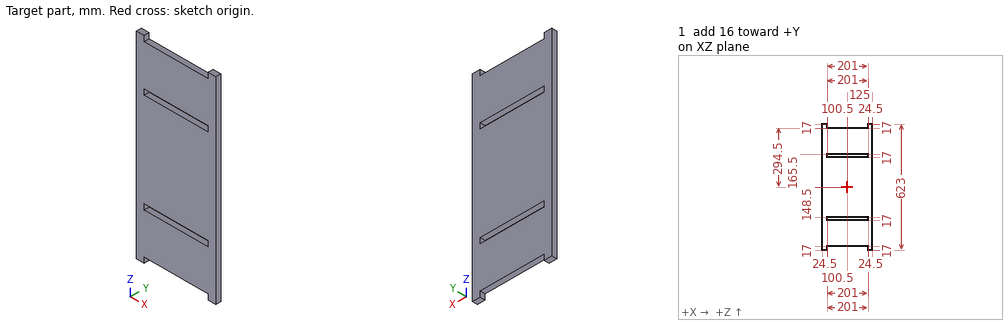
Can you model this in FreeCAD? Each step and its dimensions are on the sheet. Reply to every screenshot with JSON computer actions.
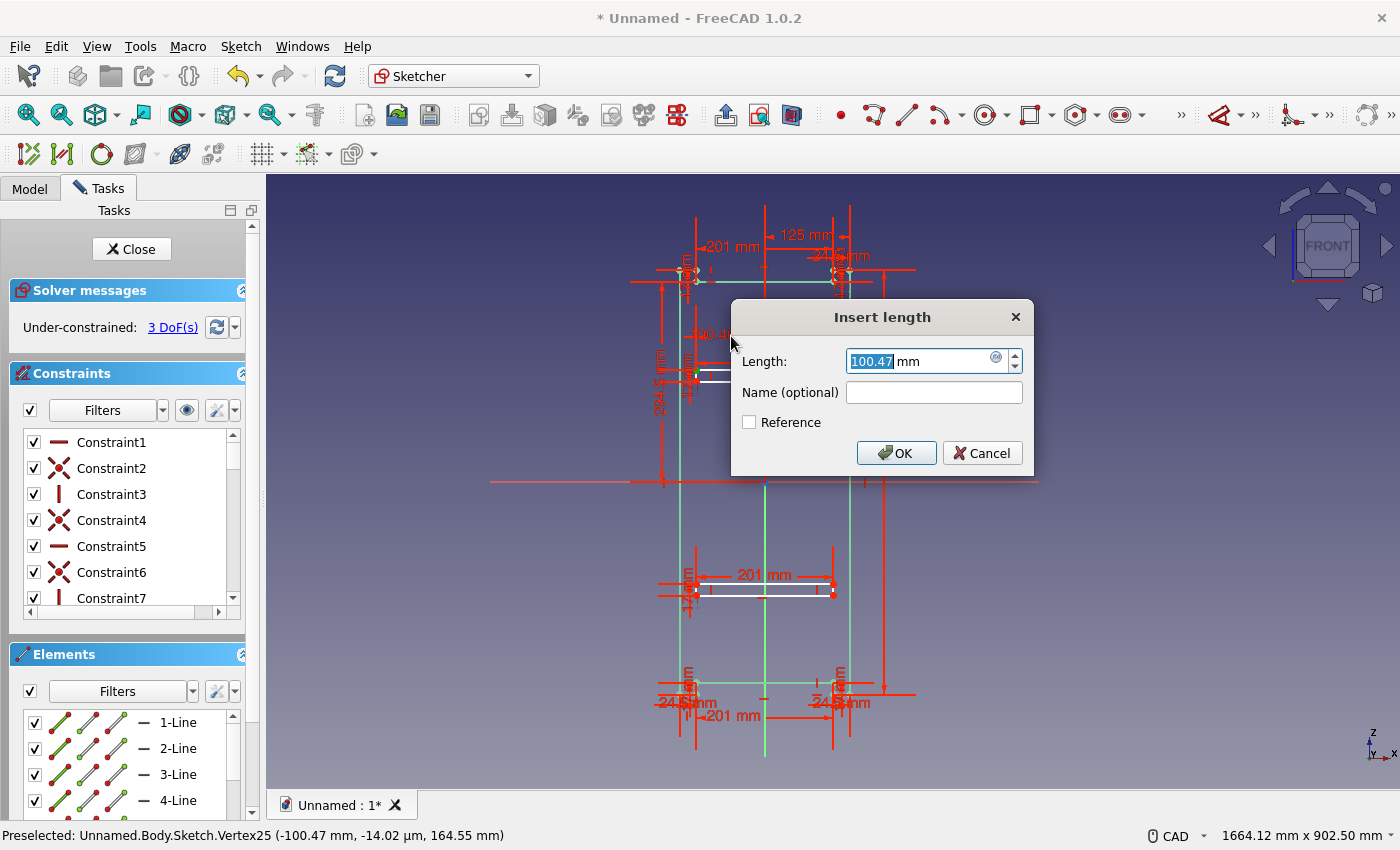
{"action": "type", "text": "100.5"}
{"action": "key", "text": "Return"}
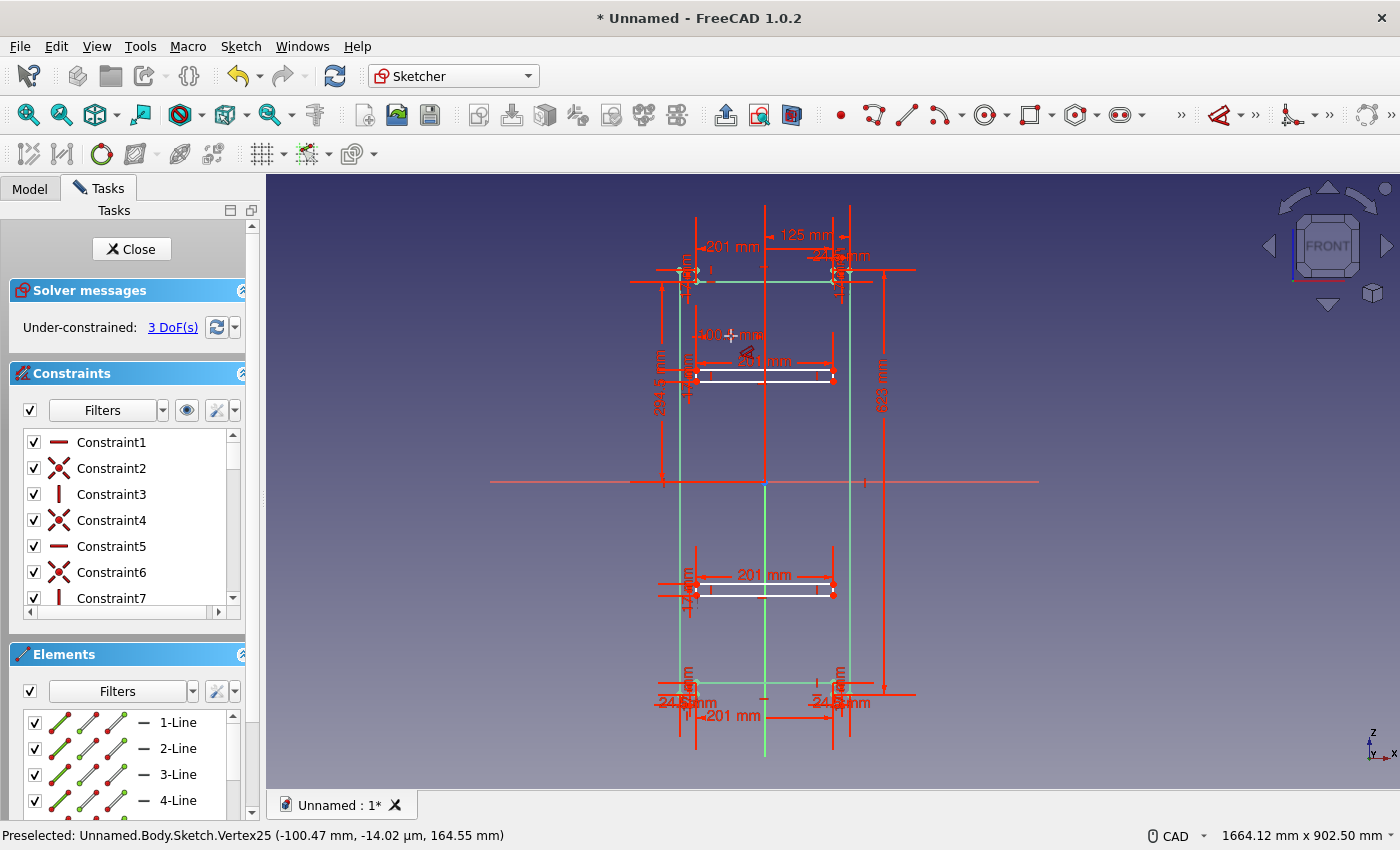
{"action": "left_click", "coordinate": [696, 370]}
{"action": "left_click", "coordinate": [662, 426]}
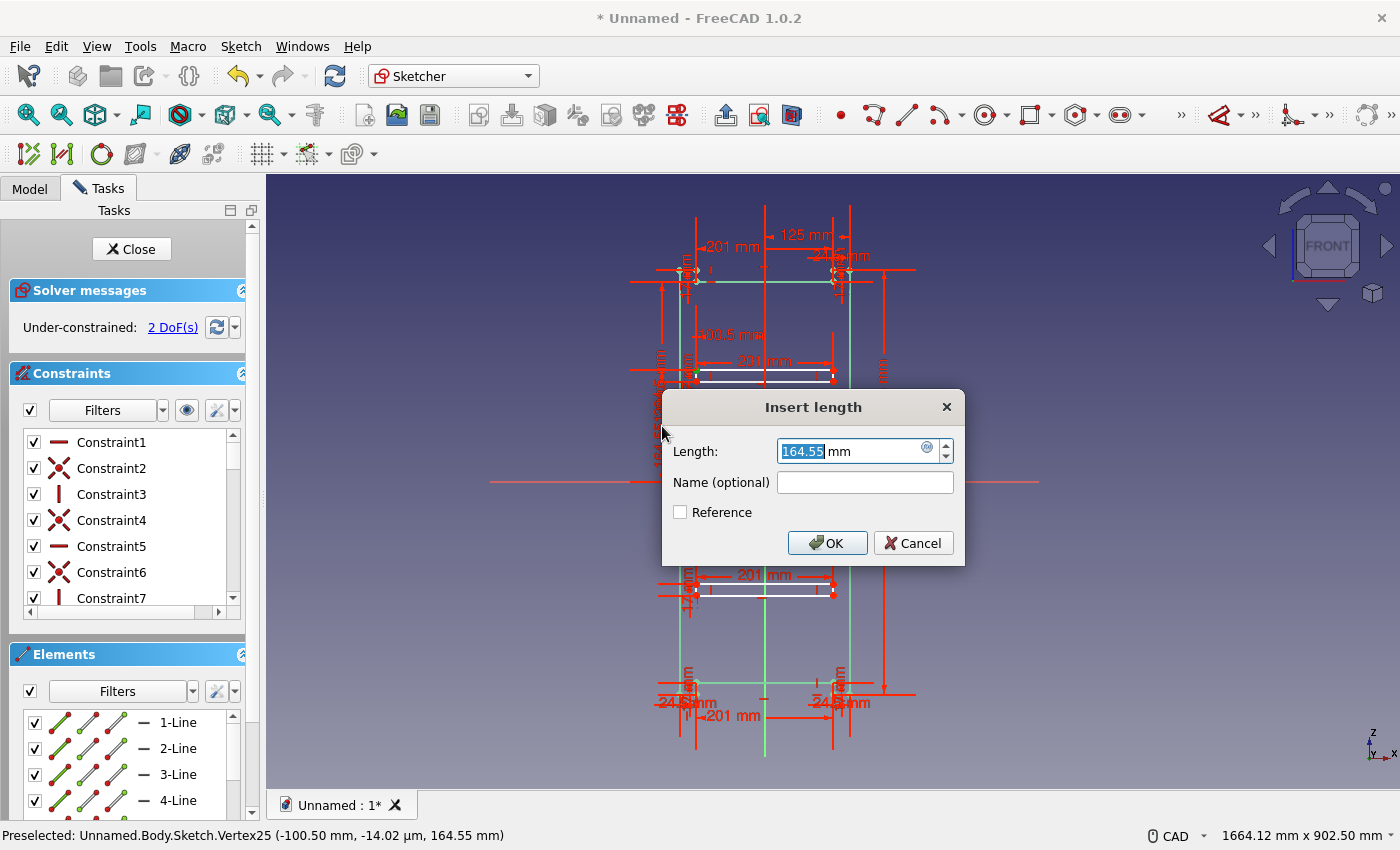
{"action": "type", "text": "165.5"}
{"action": "key", "text": "Return"}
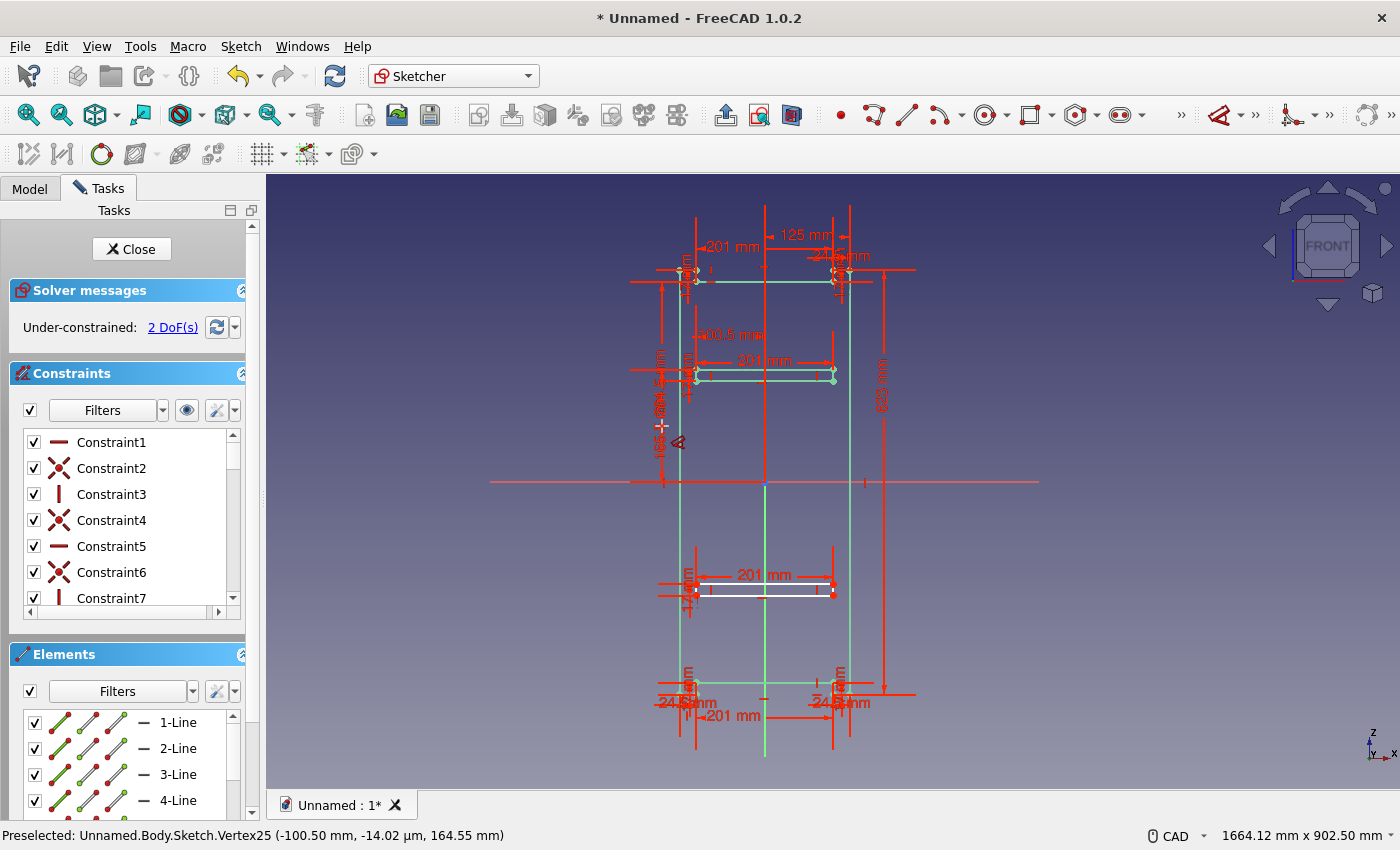
{"action": "left_click", "coordinate": [696, 584]}
{"action": "left_click", "coordinate": [731, 618]}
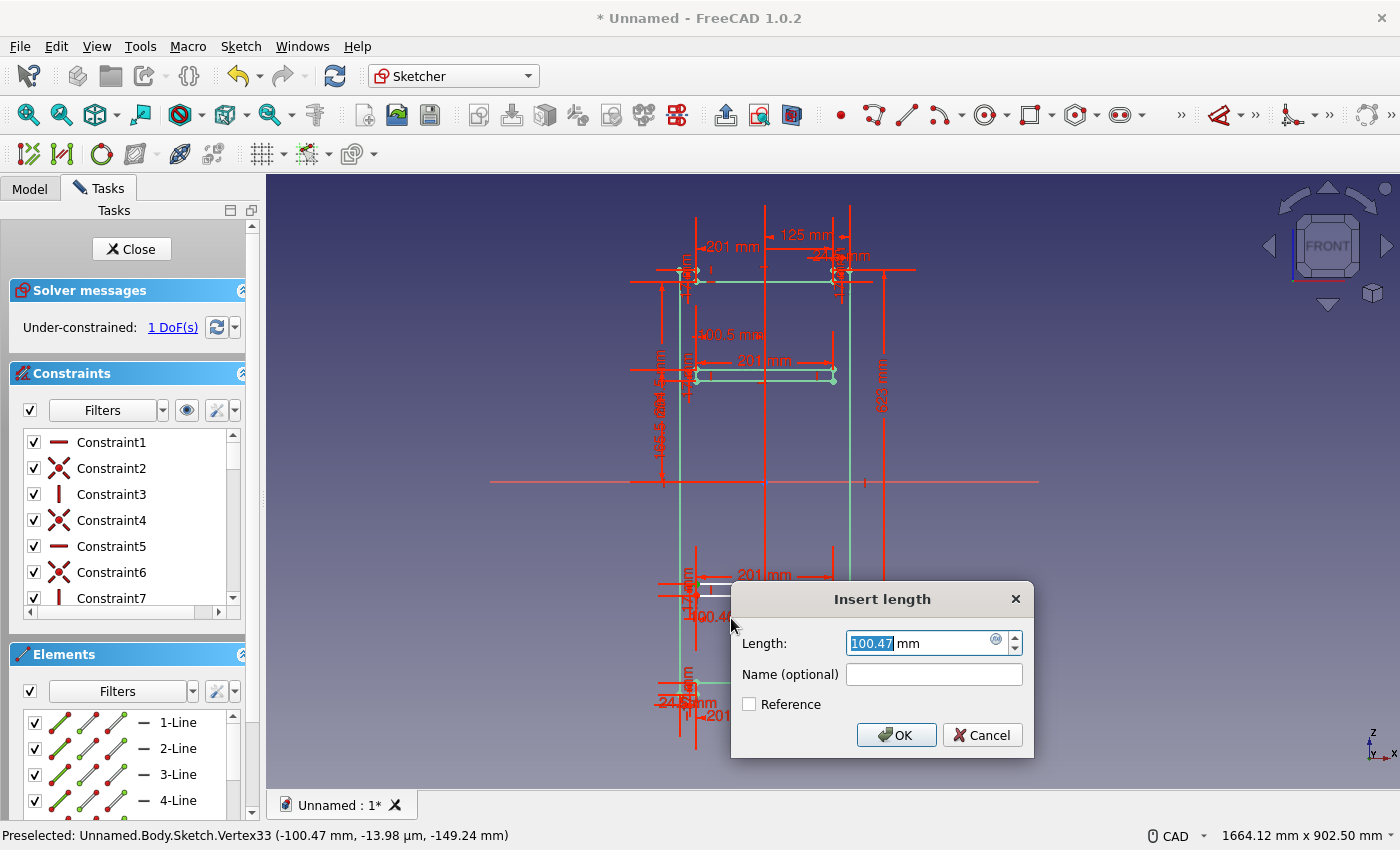
{"action": "type", "text": "100.5"}
{"action": "key", "text": "Return"}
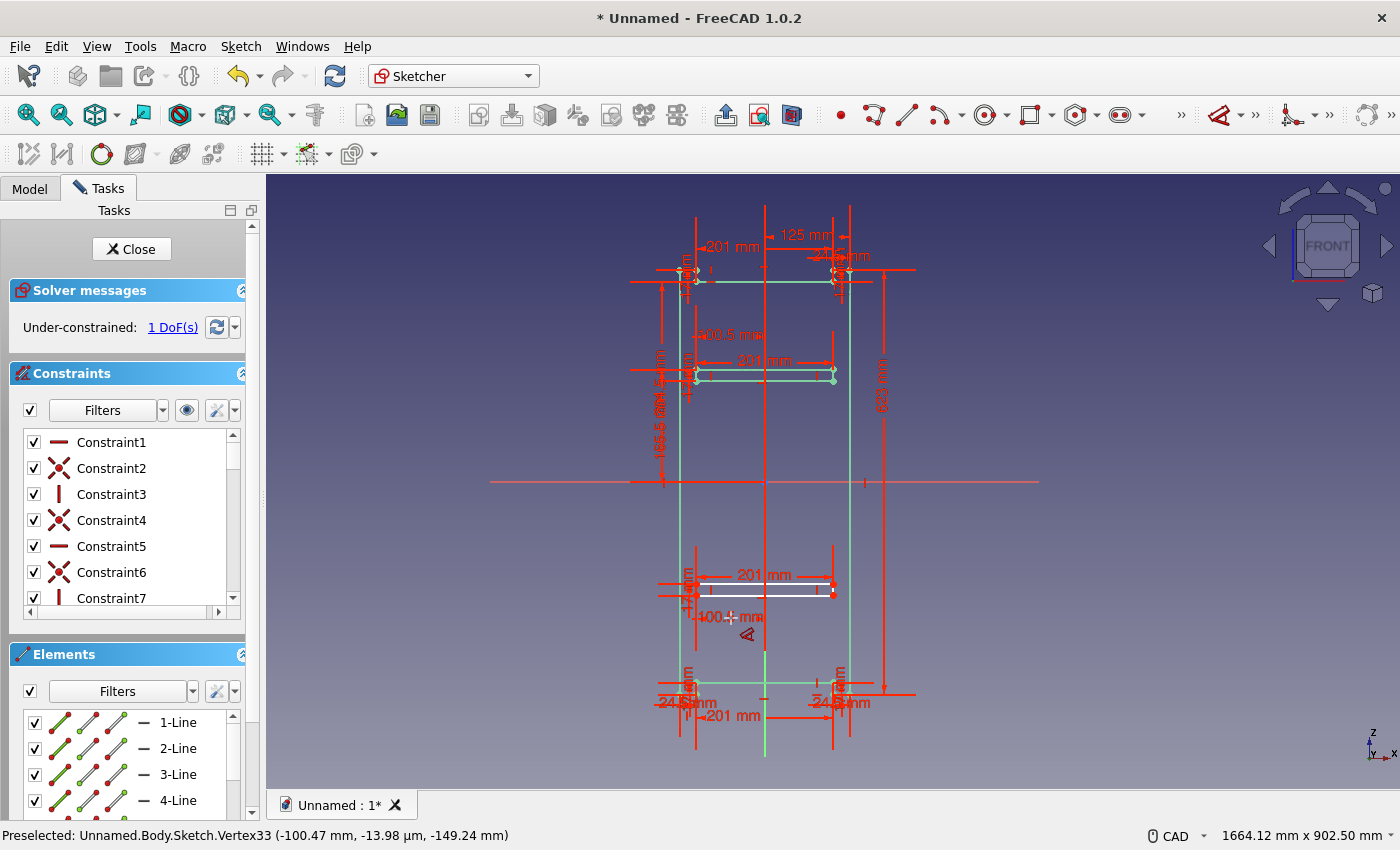
{"action": "left_click", "coordinate": [696, 584]}
{"action": "left_click", "coordinate": [662, 533]}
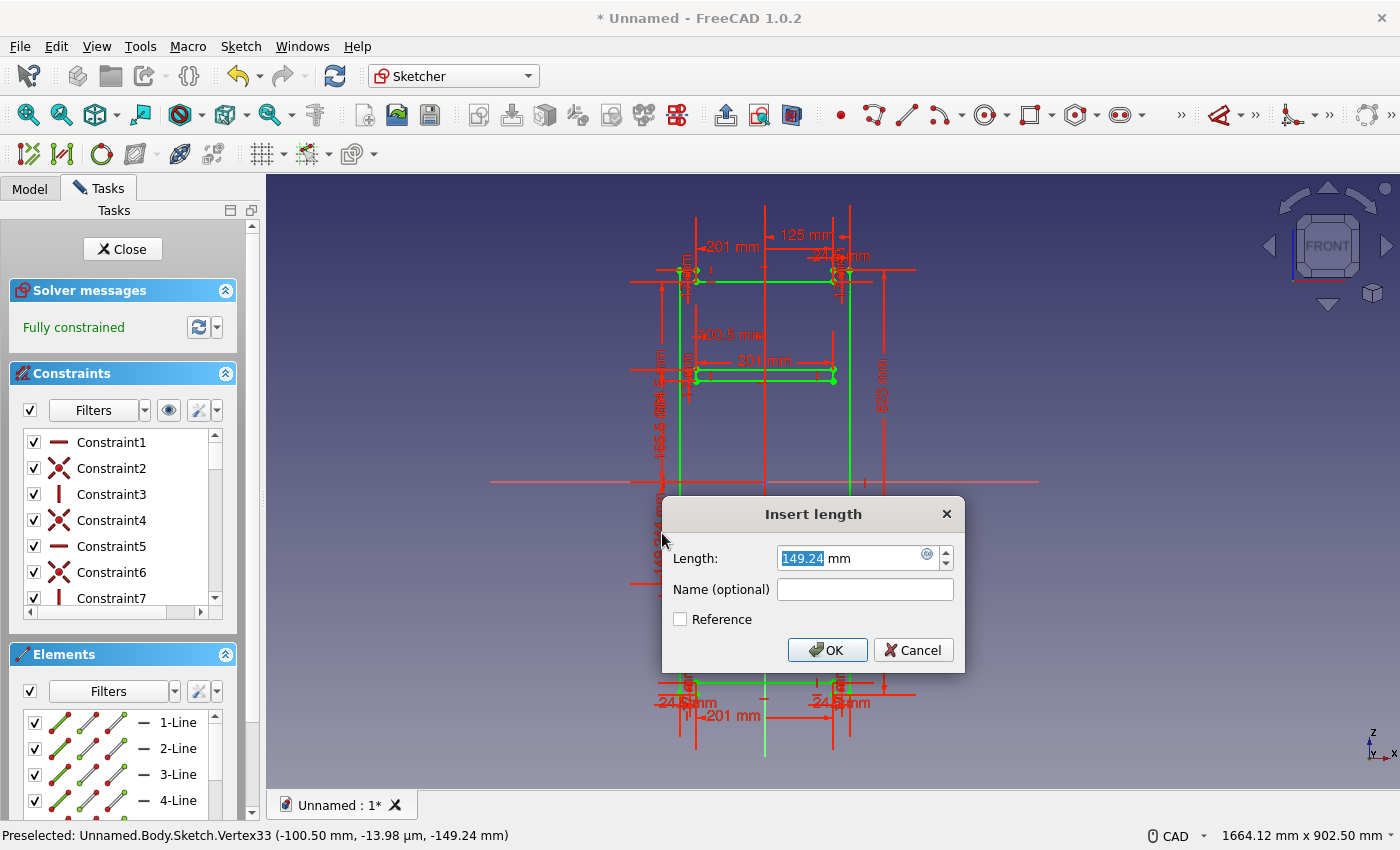
{"action": "type", "text": "148.5"}
{"action": "key", "text": "Return"}
{"action": "key", "text": "Escape"}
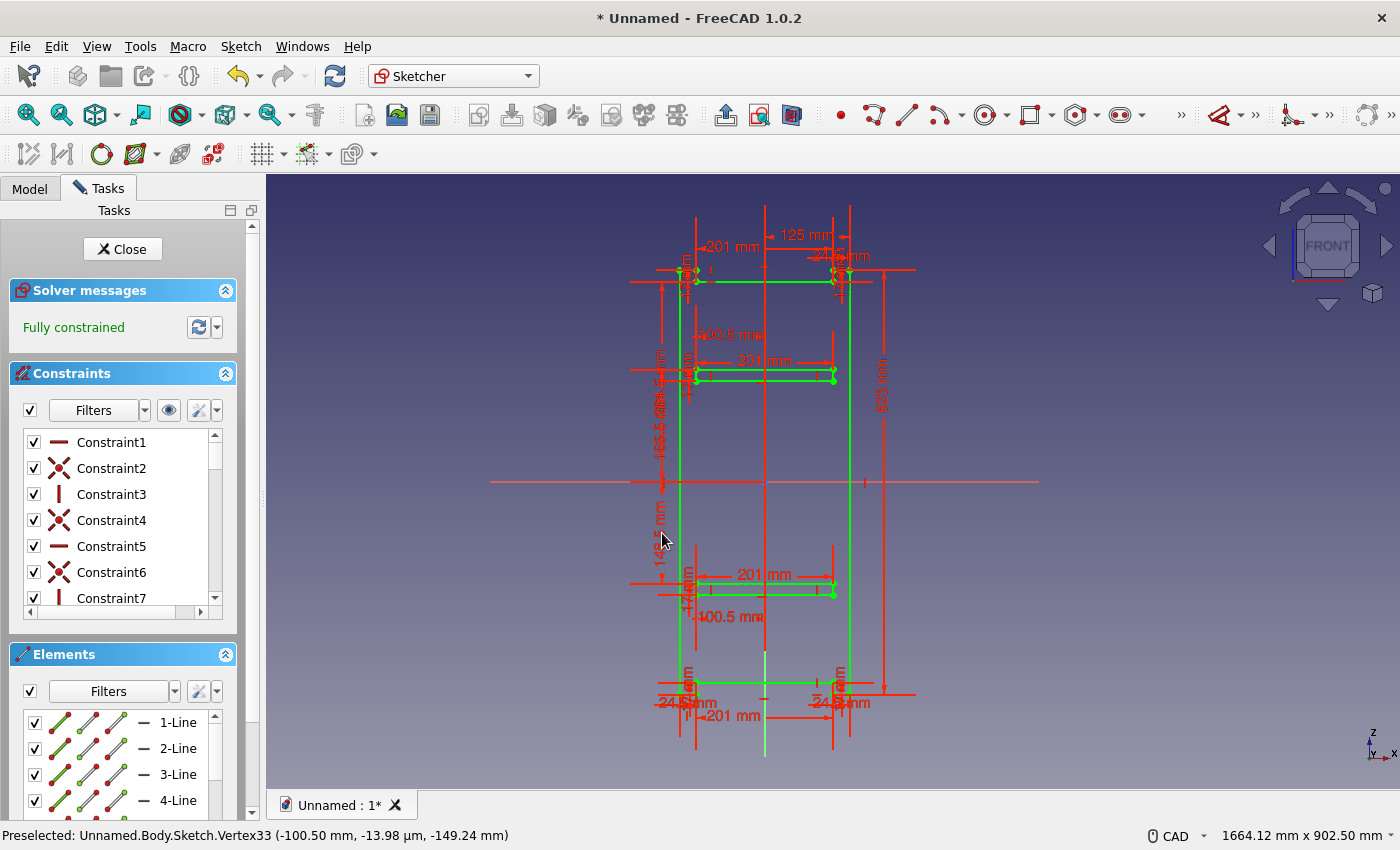
{"action": "left_click", "coordinate": [123, 249]}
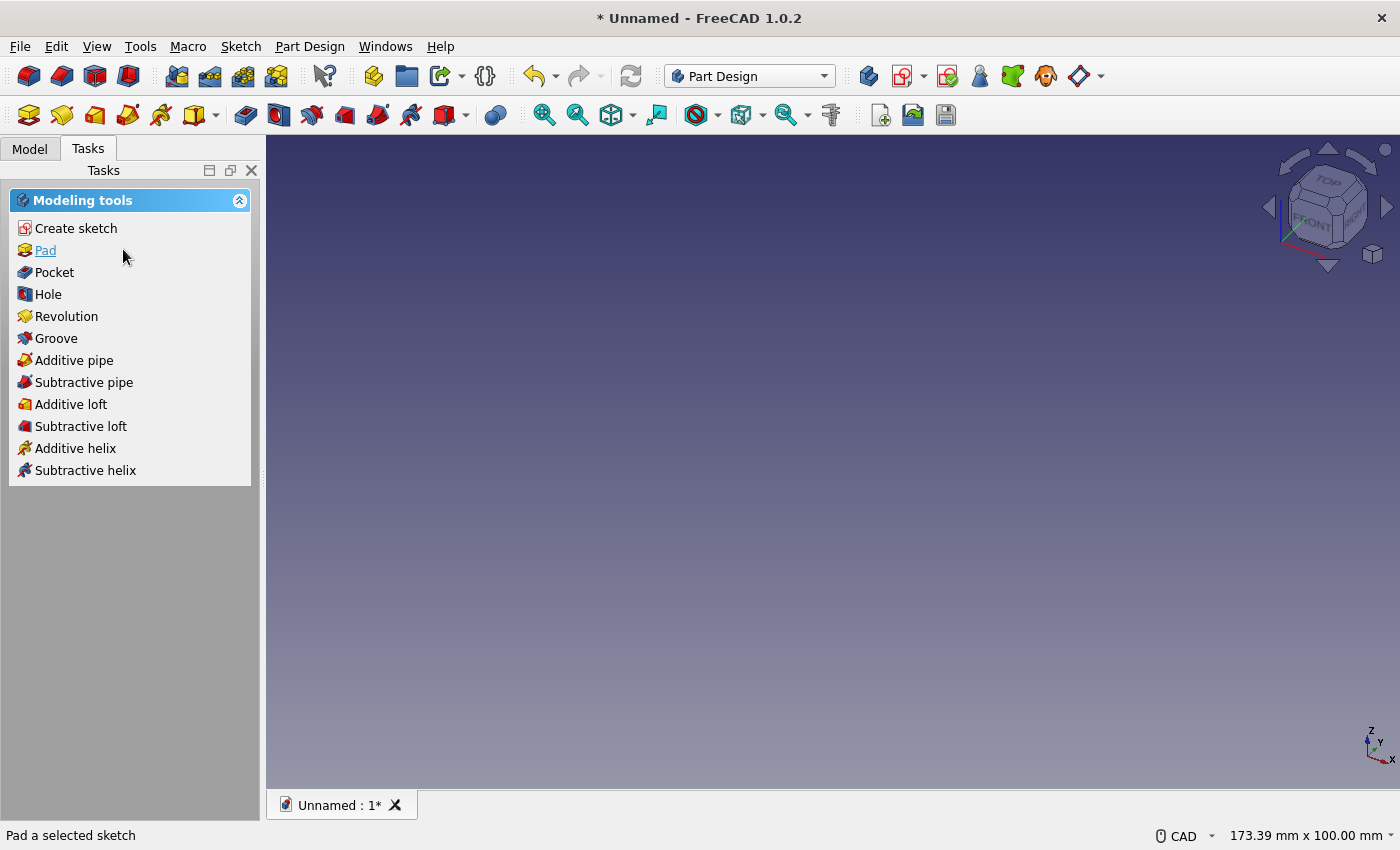
{"action": "left_click", "coordinate": [29, 116]}